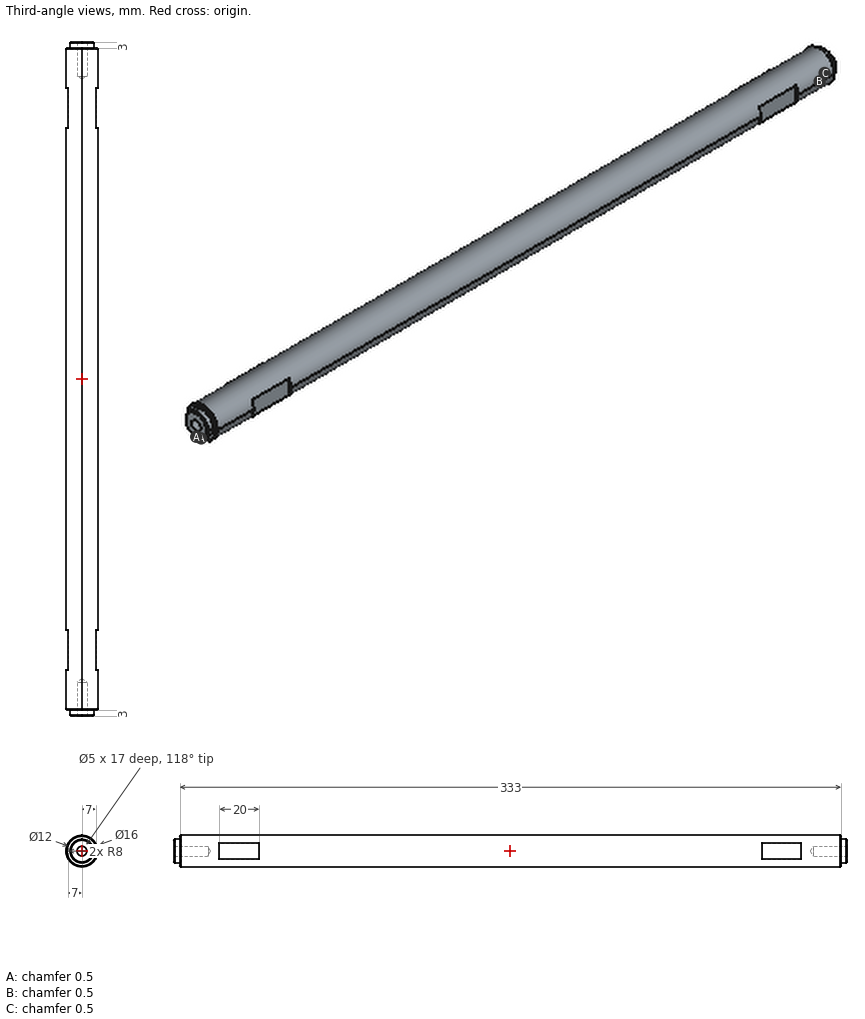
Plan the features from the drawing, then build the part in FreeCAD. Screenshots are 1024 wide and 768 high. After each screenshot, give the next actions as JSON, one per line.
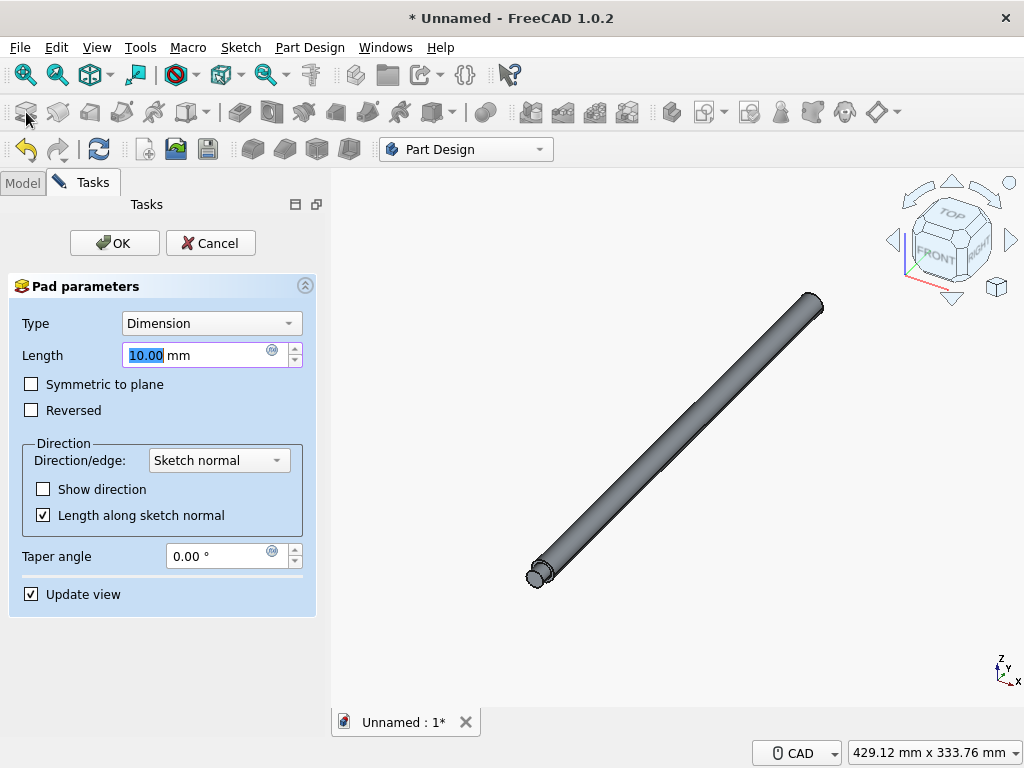
{"action": "type", "text": "3"}
{"action": "key", "text": "Tab"}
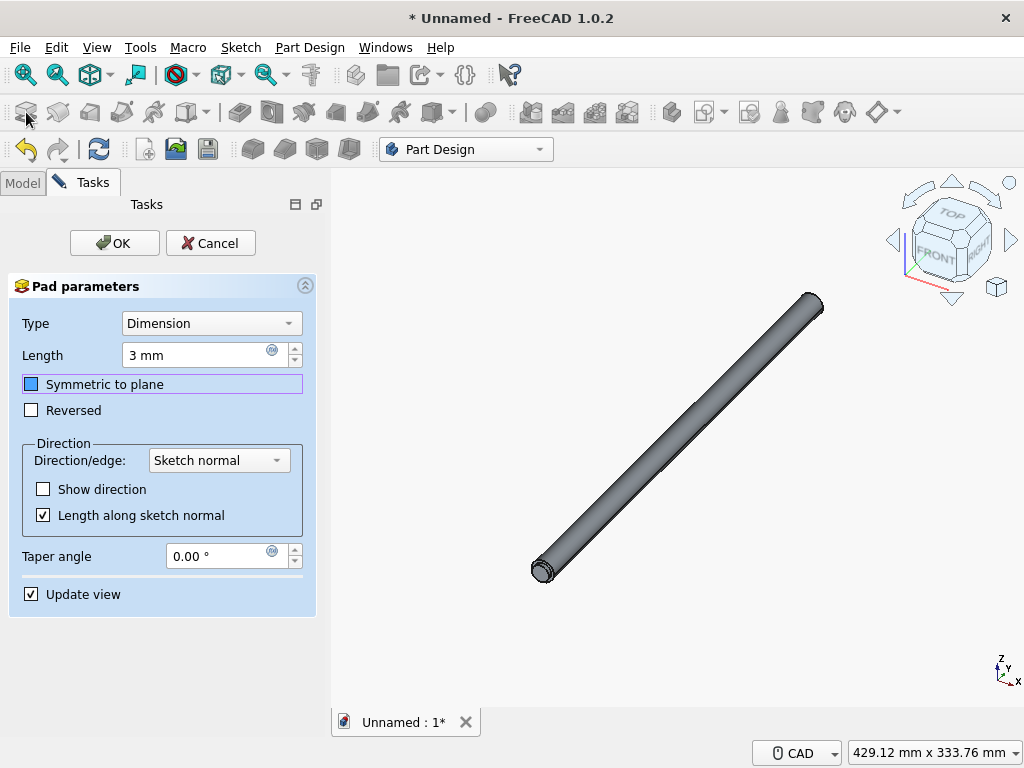
{"action": "left_click", "coordinate": [115, 243]}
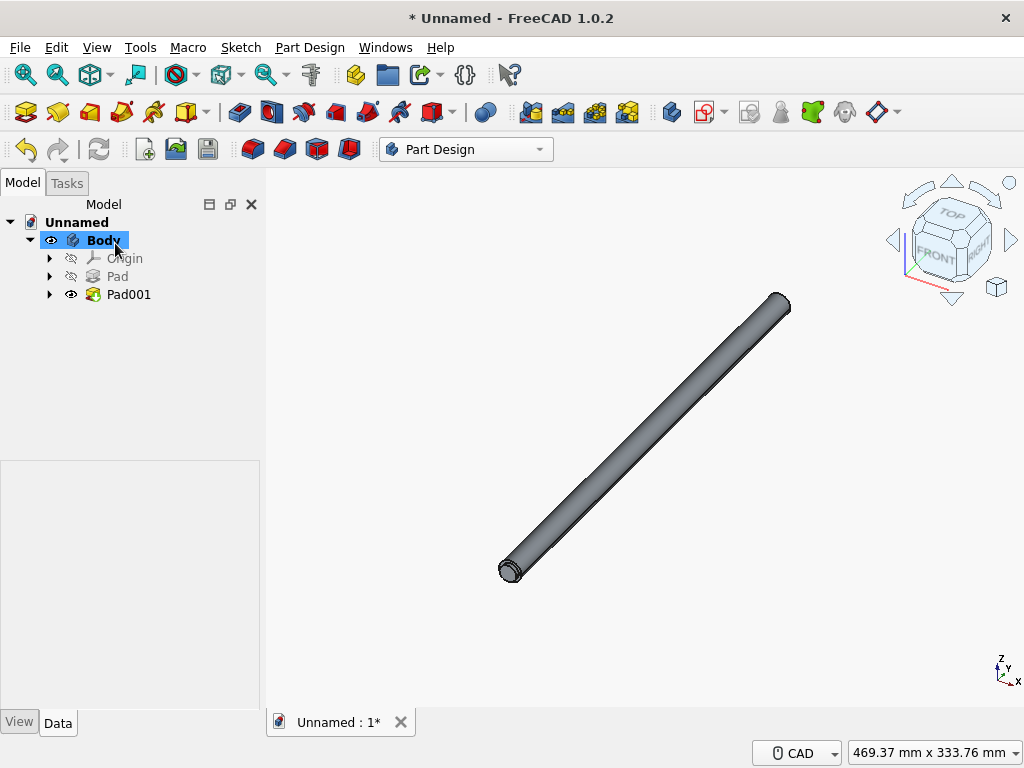
{"action": "left_click", "coordinate": [500, 570]}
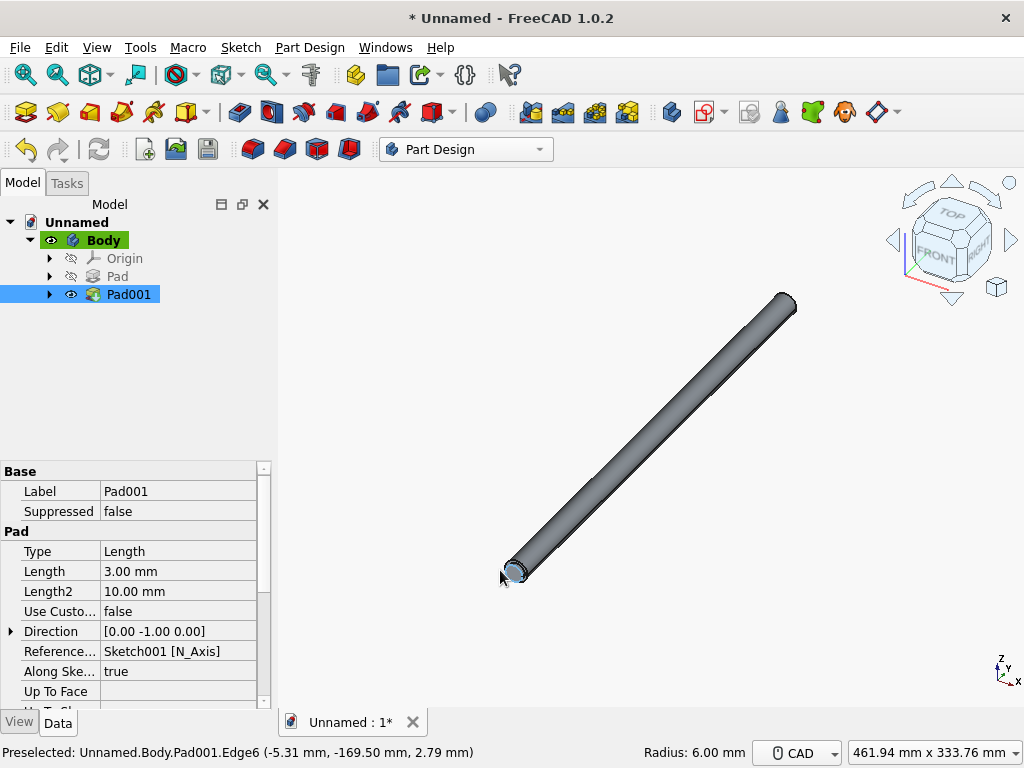
{"action": "key", "text": "0"}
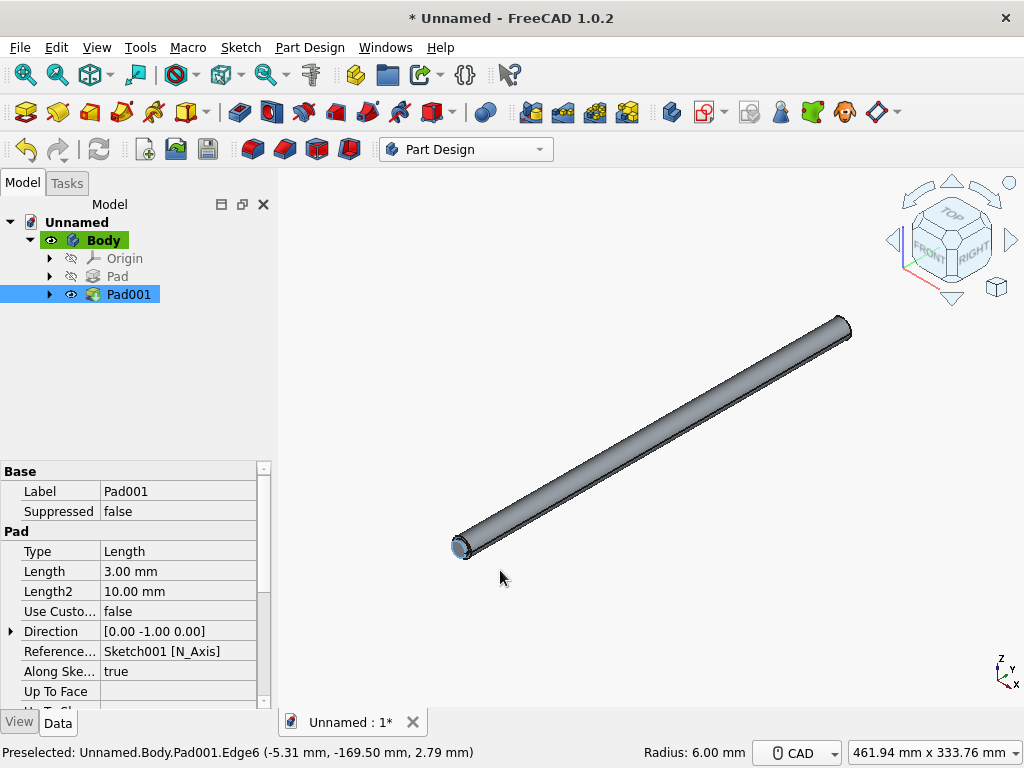
{"action": "left_click", "coordinate": [465, 538], "text": "ctrl"}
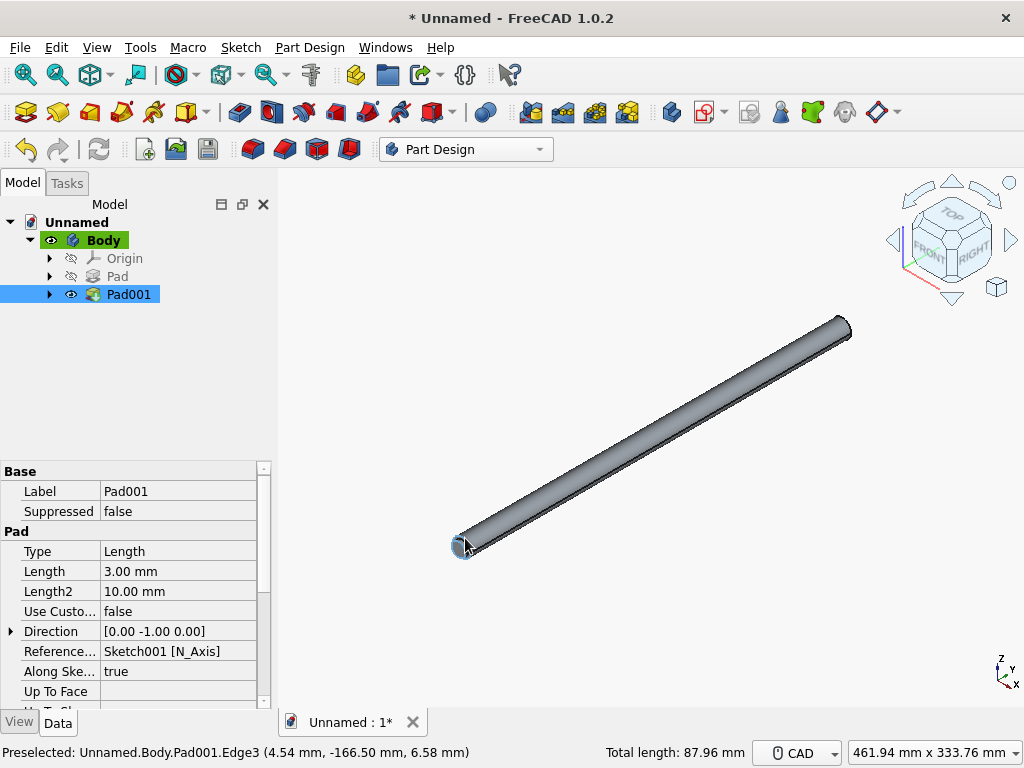
{"action": "left_click", "coordinate": [286, 150]}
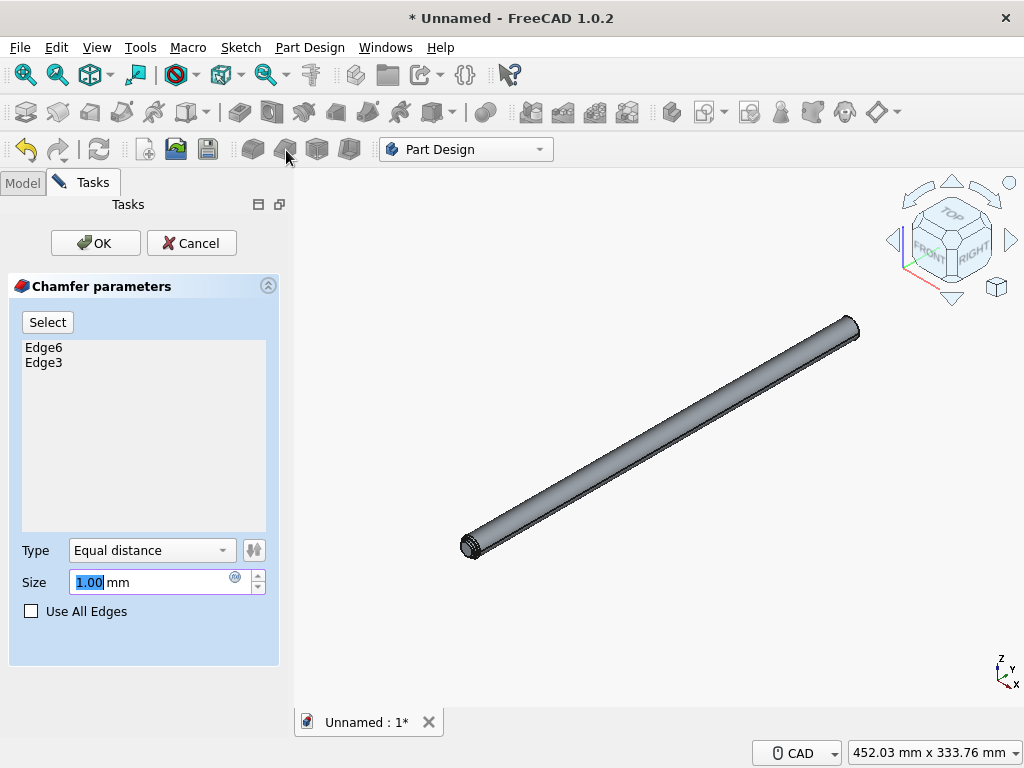
{"action": "type", "text": "0.5"}
{"action": "key", "text": "Tab"}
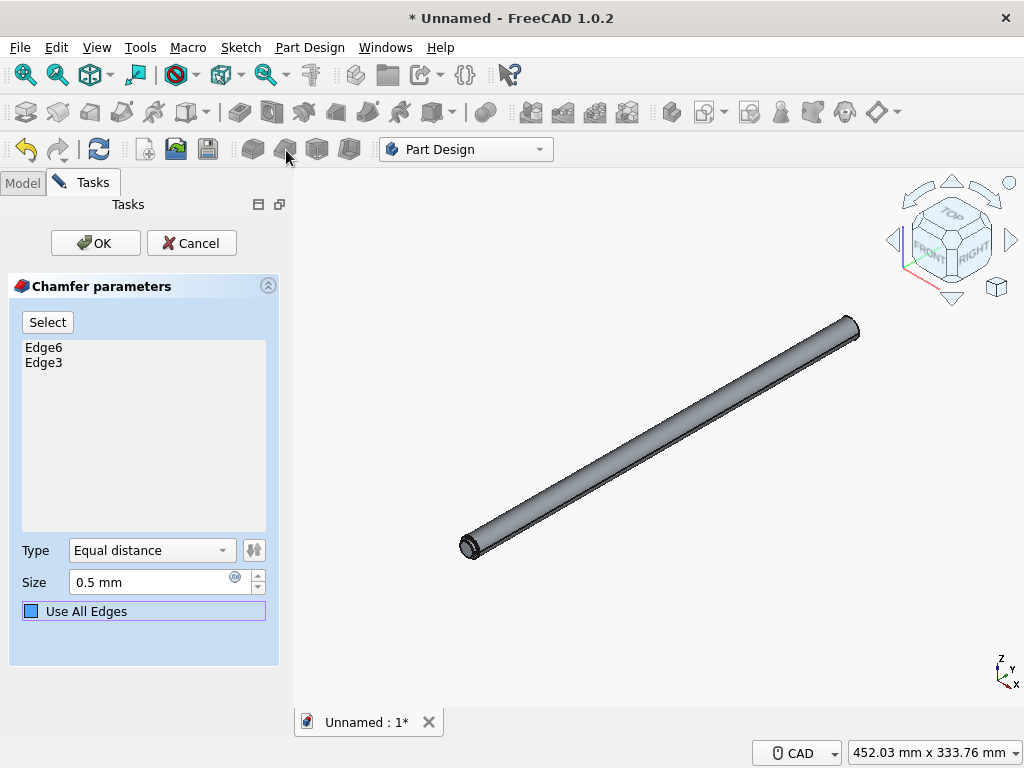
{"action": "left_click", "coordinate": [96, 243]}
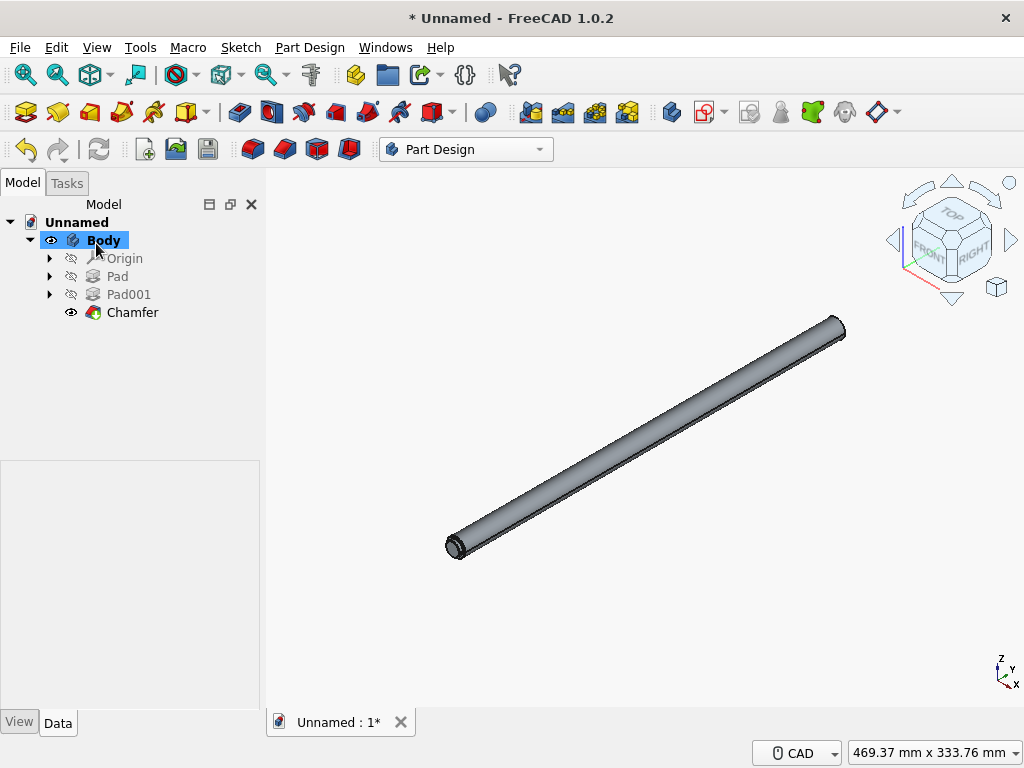
{"action": "left_click", "coordinate": [50, 258]}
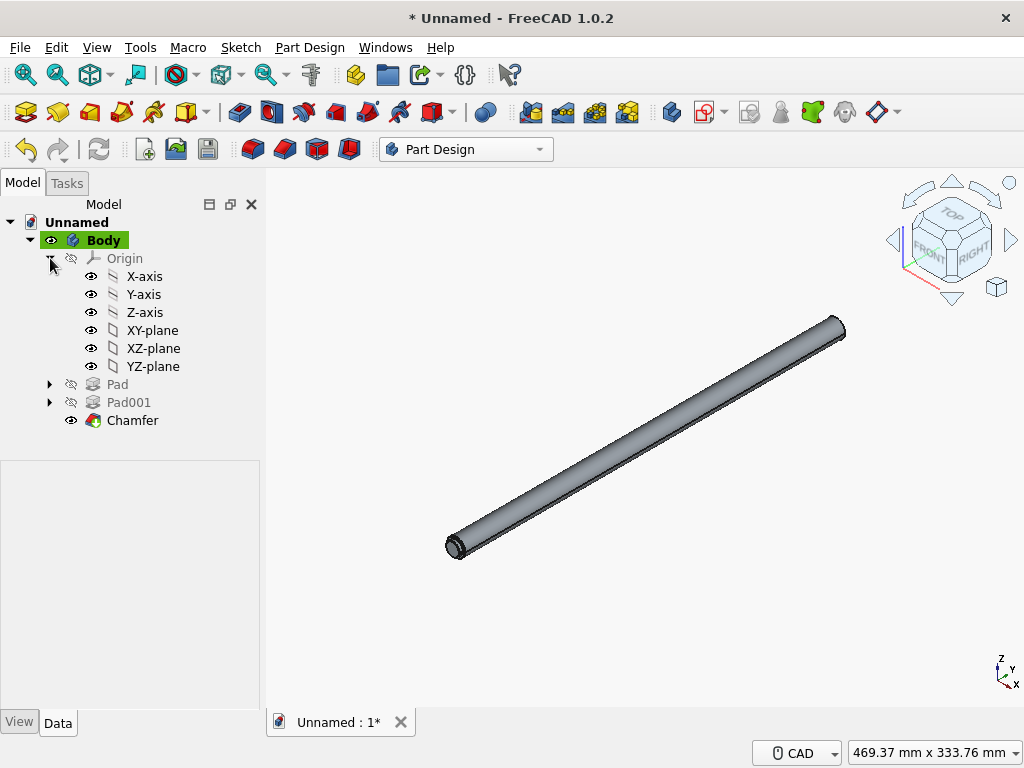
{"action": "left_click", "coordinate": [136, 348]}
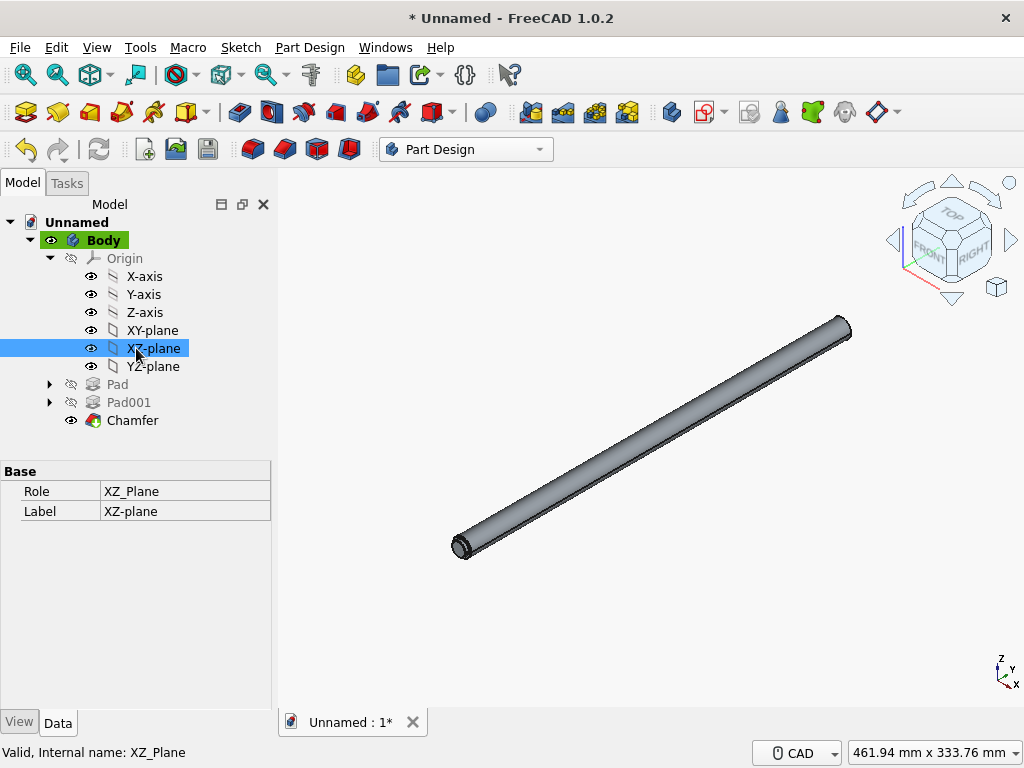
{"action": "left_click", "coordinate": [878, 112]}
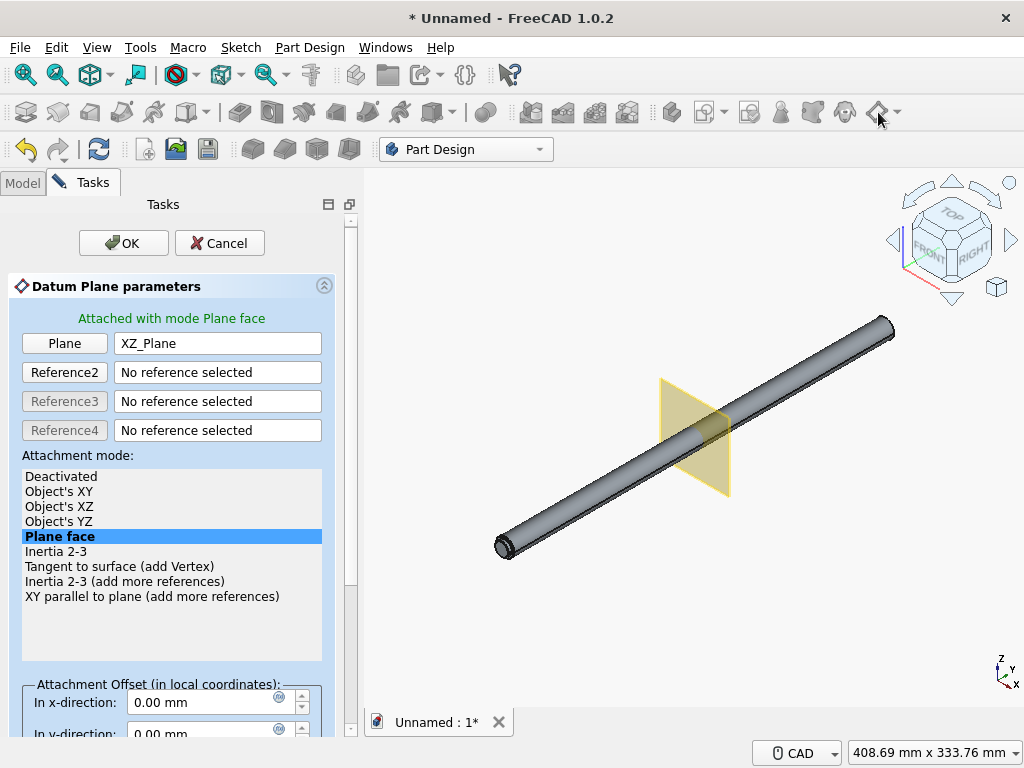
{"action": "scroll", "coordinate": [351, 475], "scroll_direction": "down", "scroll_amount": 2}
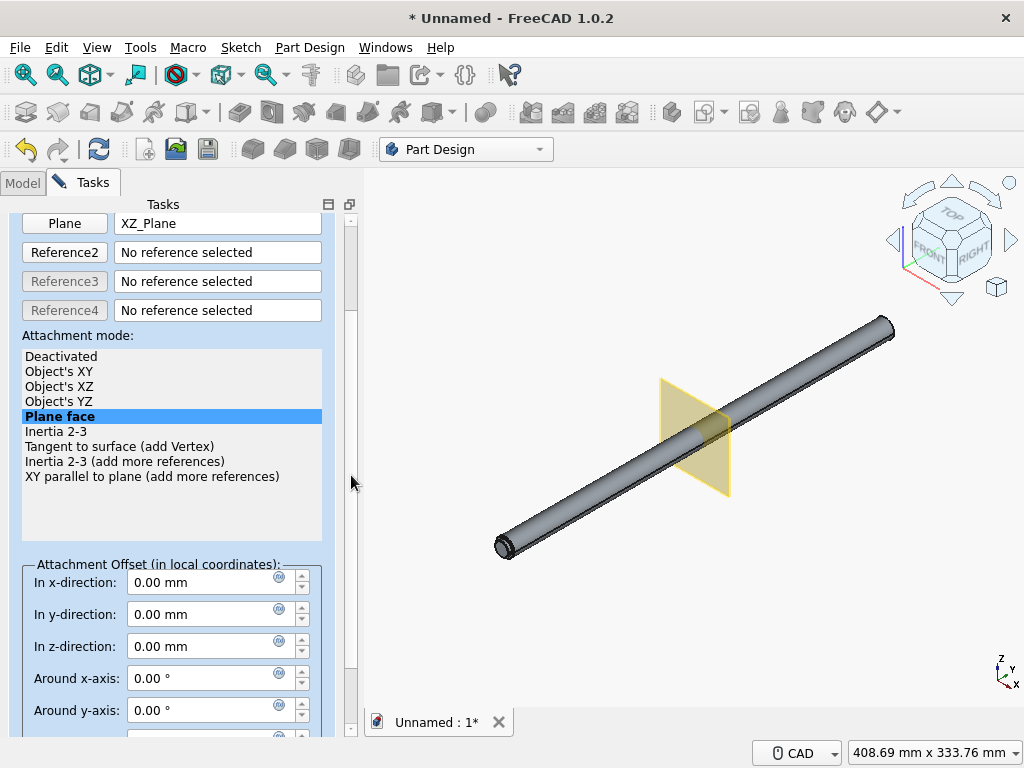
{"action": "triple_click", "coordinate": [210, 646]}